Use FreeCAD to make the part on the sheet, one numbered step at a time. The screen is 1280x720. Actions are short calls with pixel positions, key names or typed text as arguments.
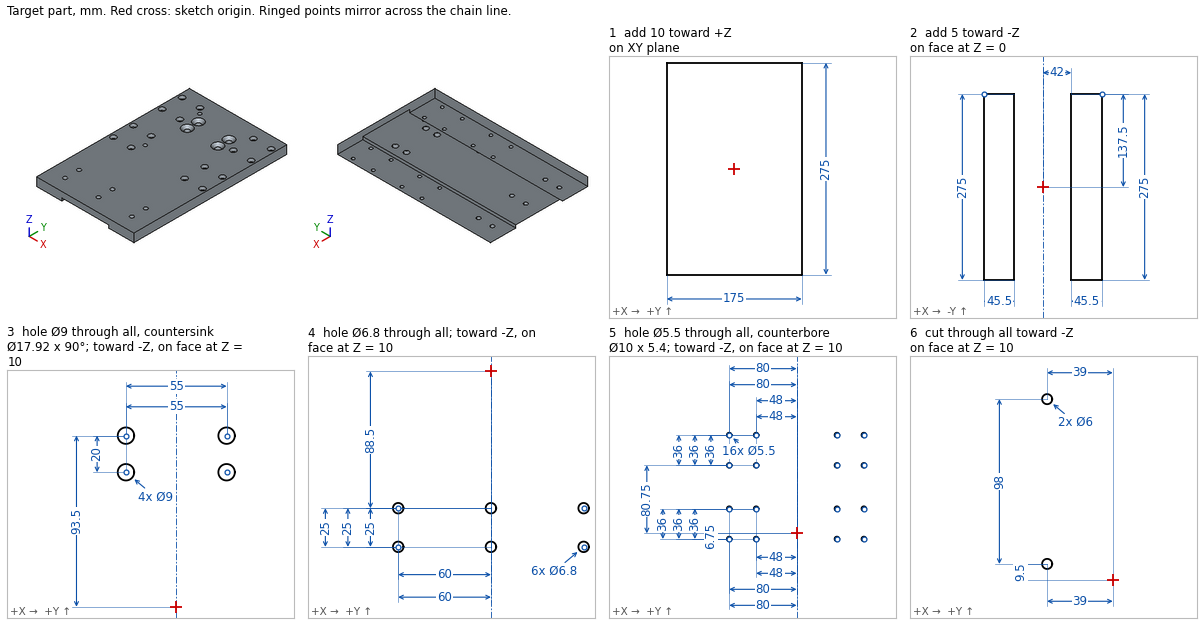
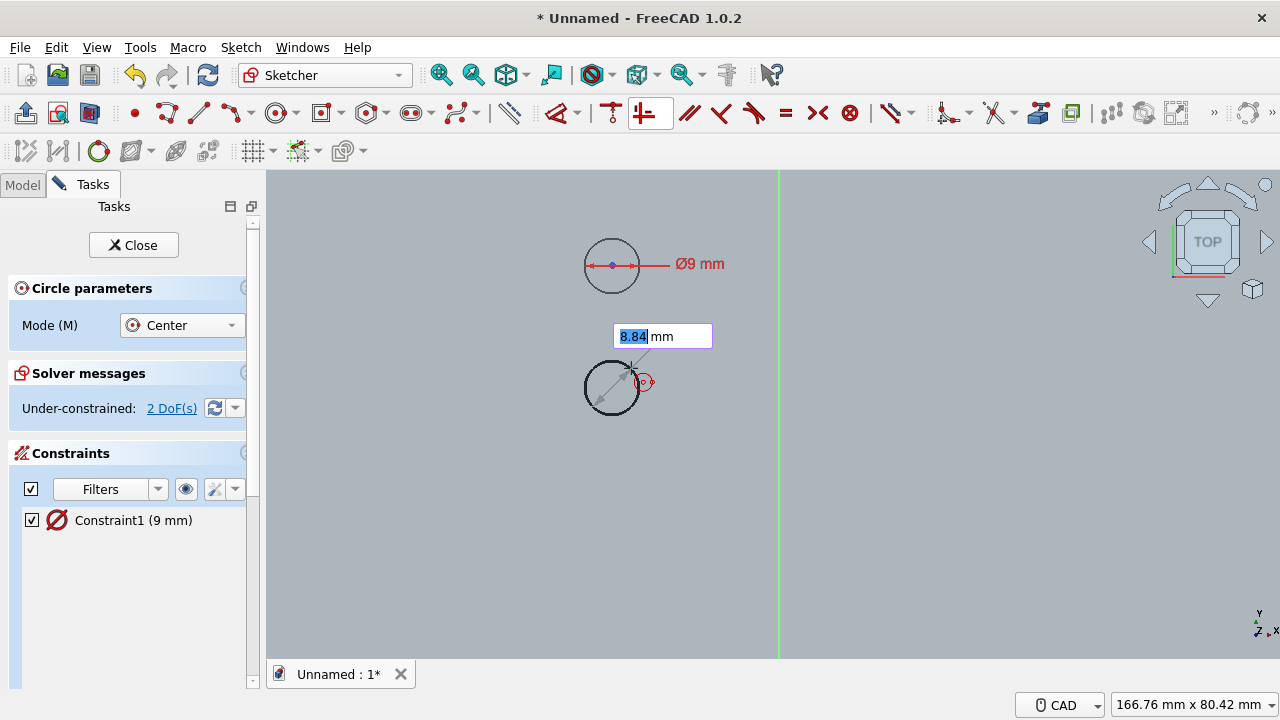
text(9)
key(Return)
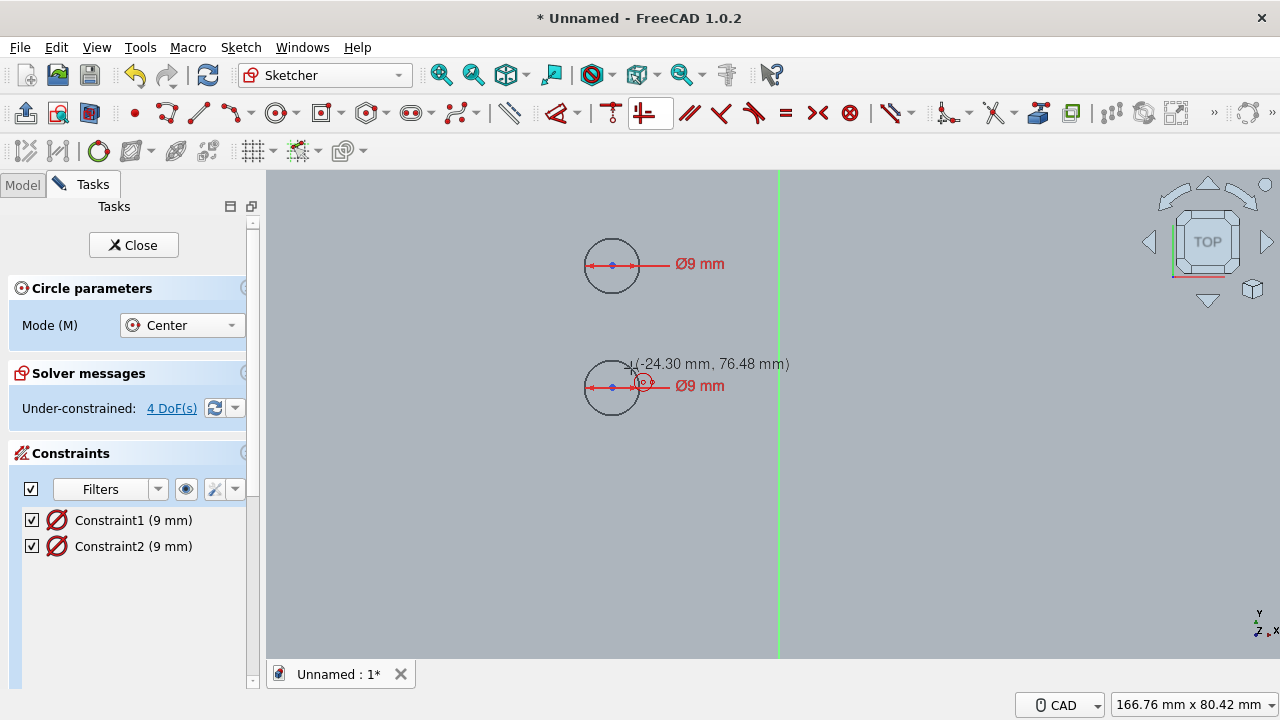
click(946, 265)
move(965, 246)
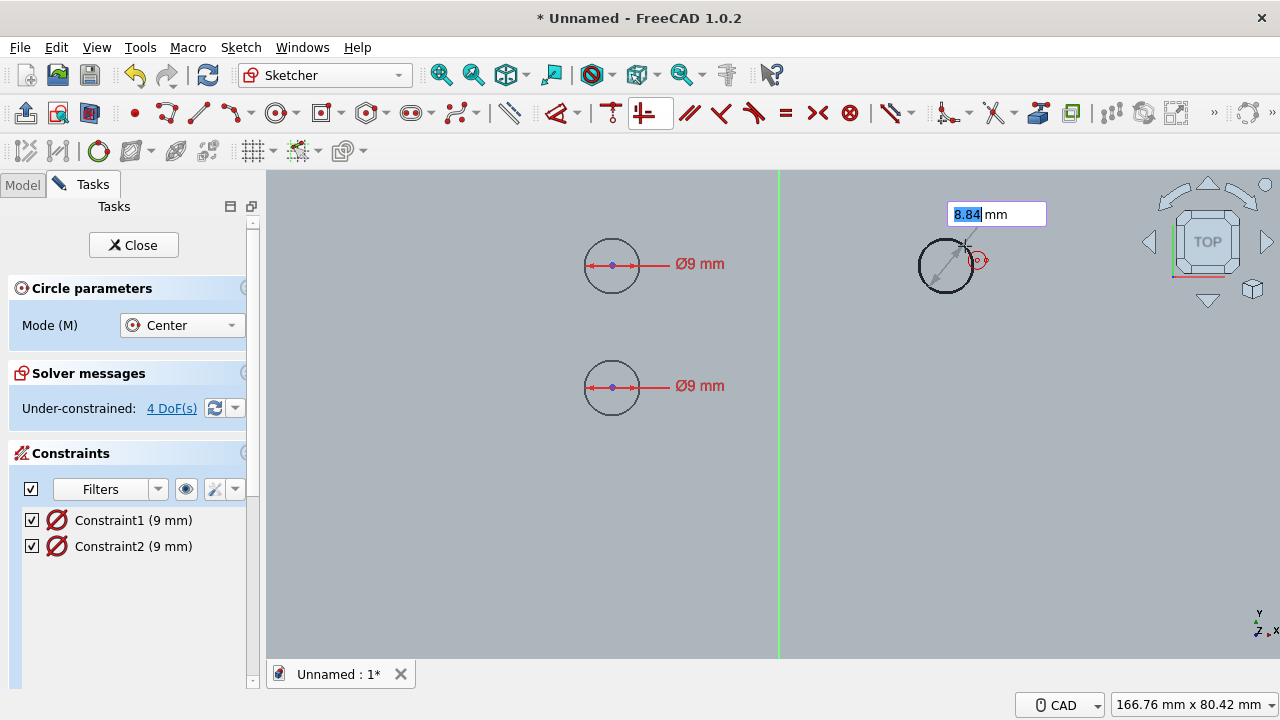
text(9)
key(Return)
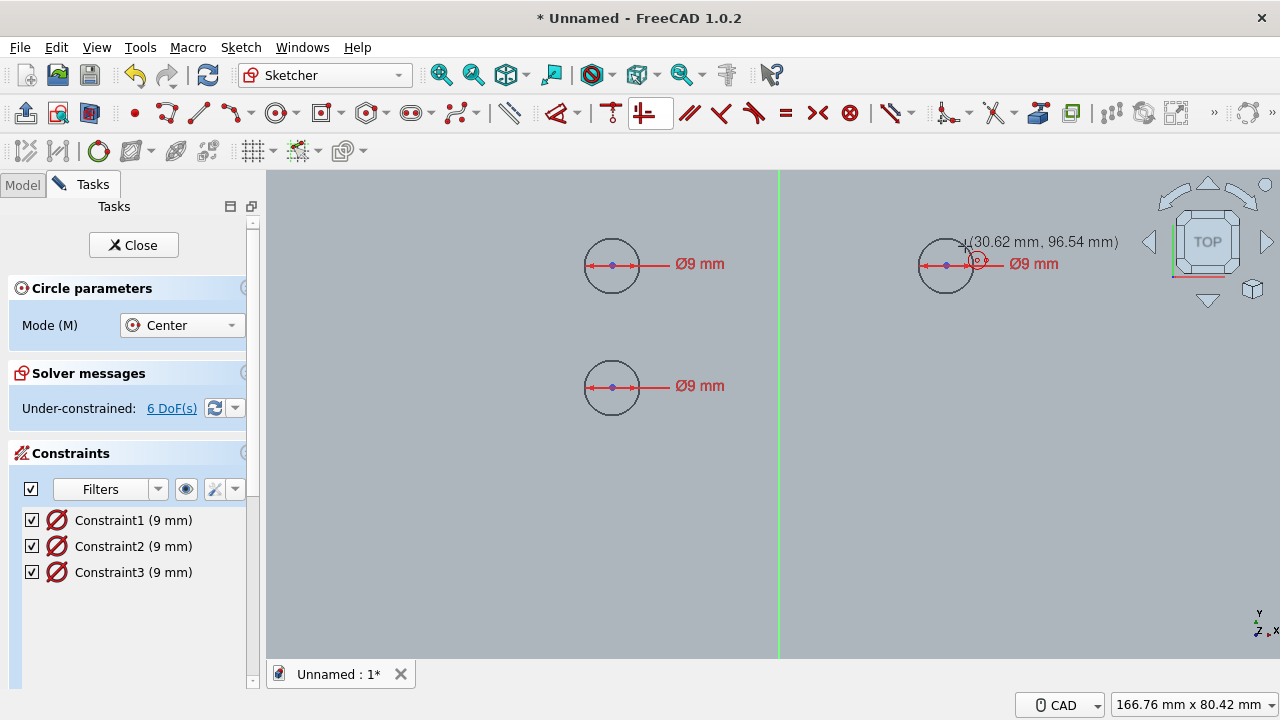
click(946, 387)
move(965, 368)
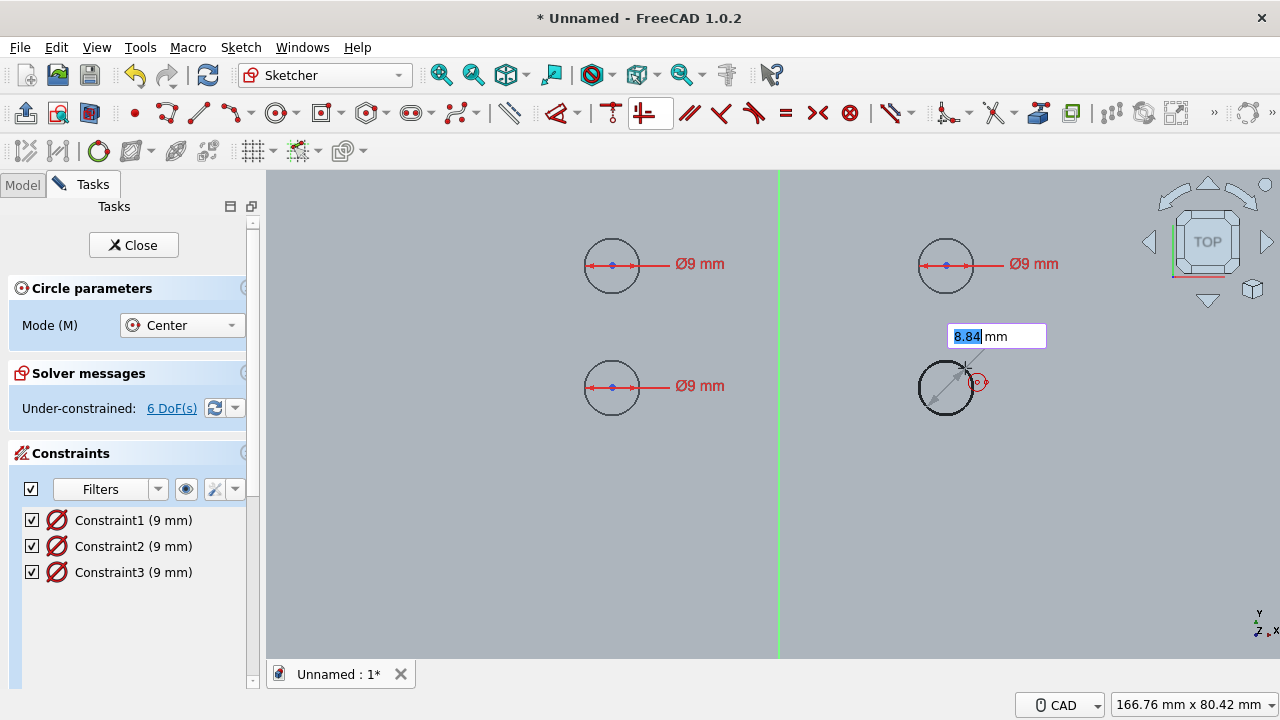
text(9)
key(Return)
key(Escape)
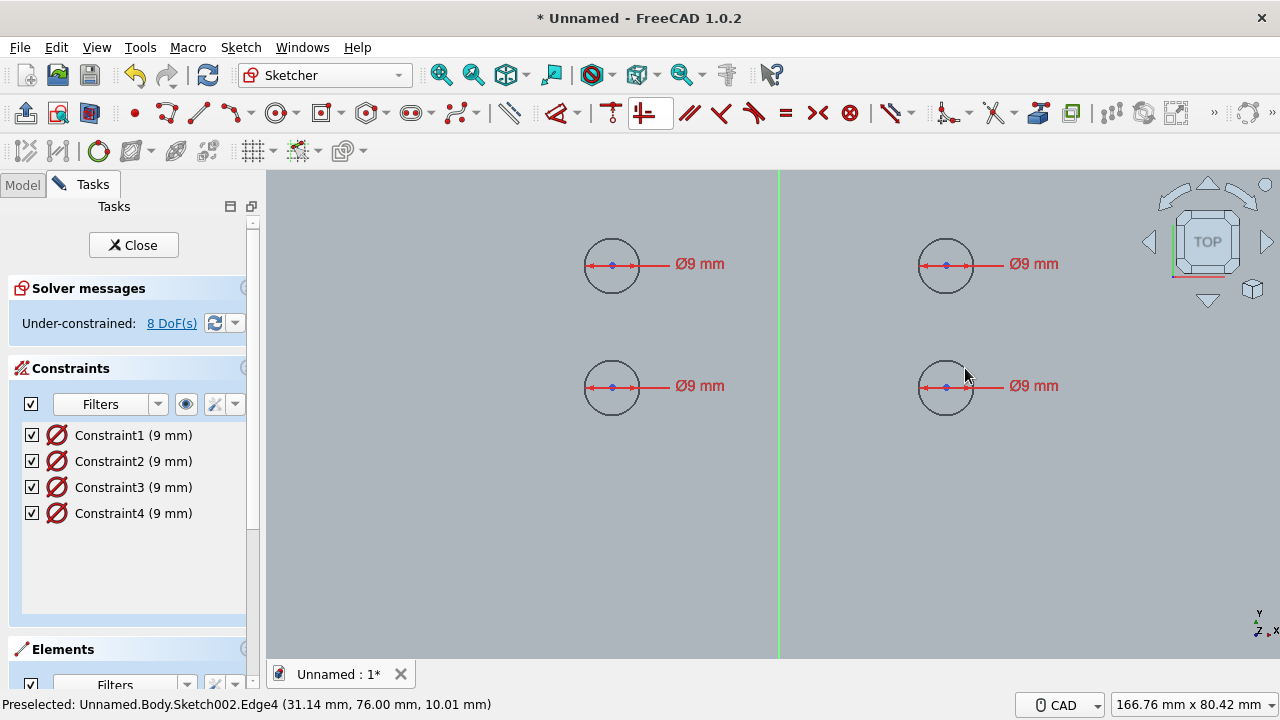
click(612, 266)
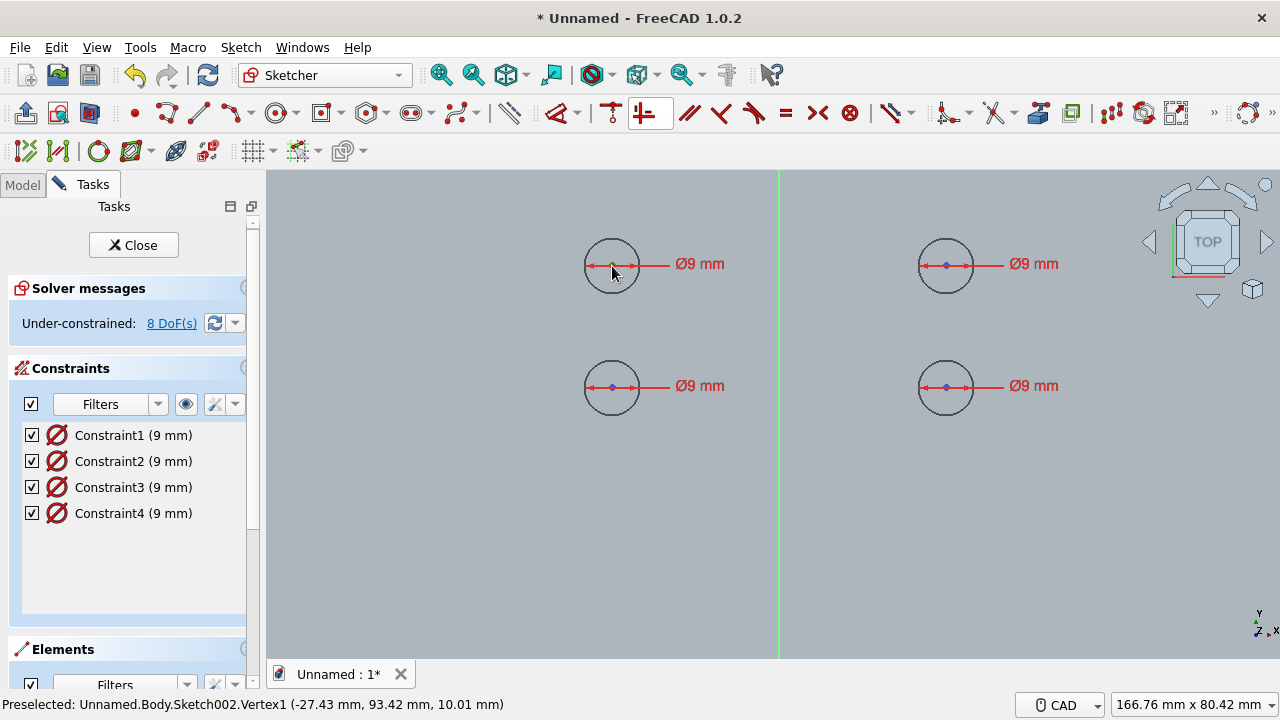
click(946, 266)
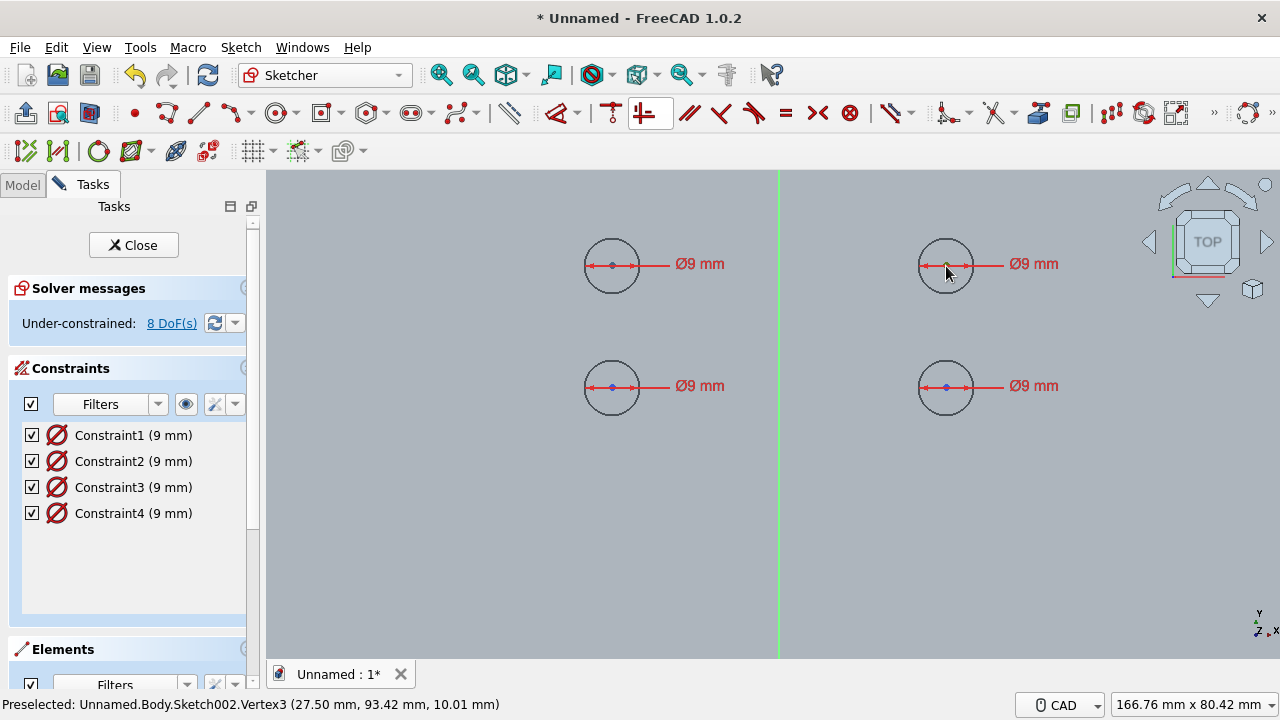
click(779, 600)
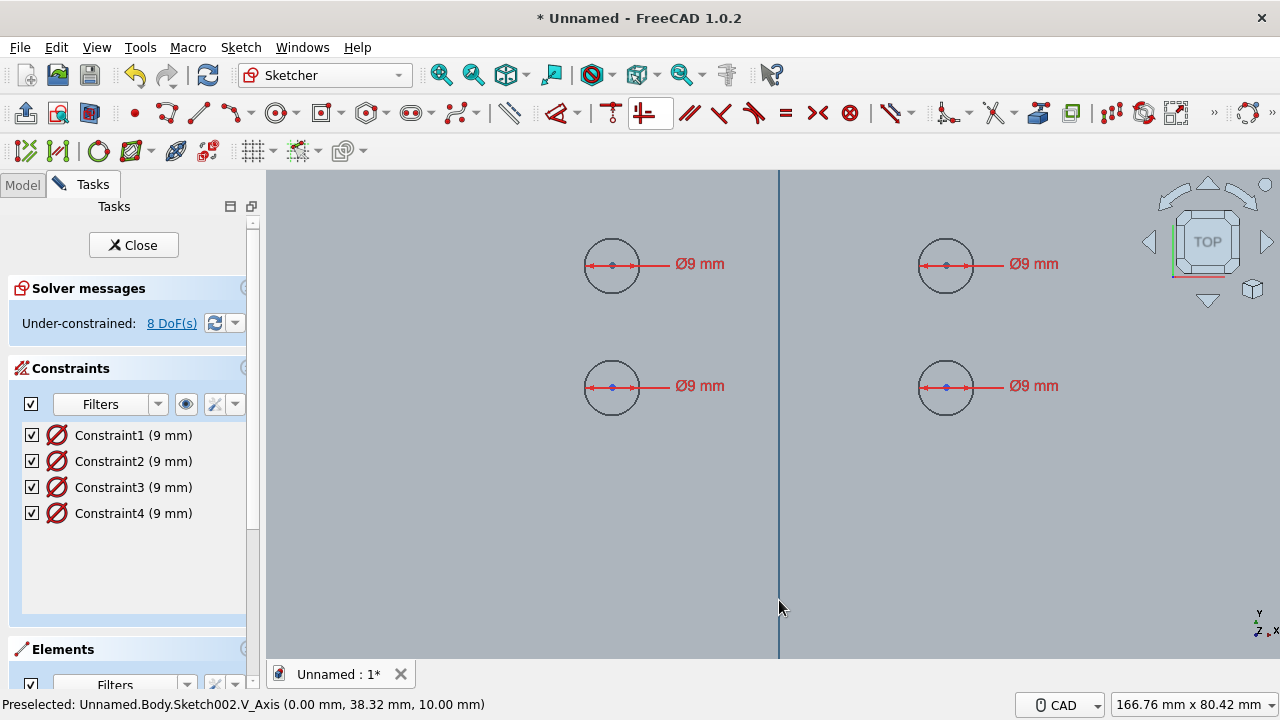
click(818, 114)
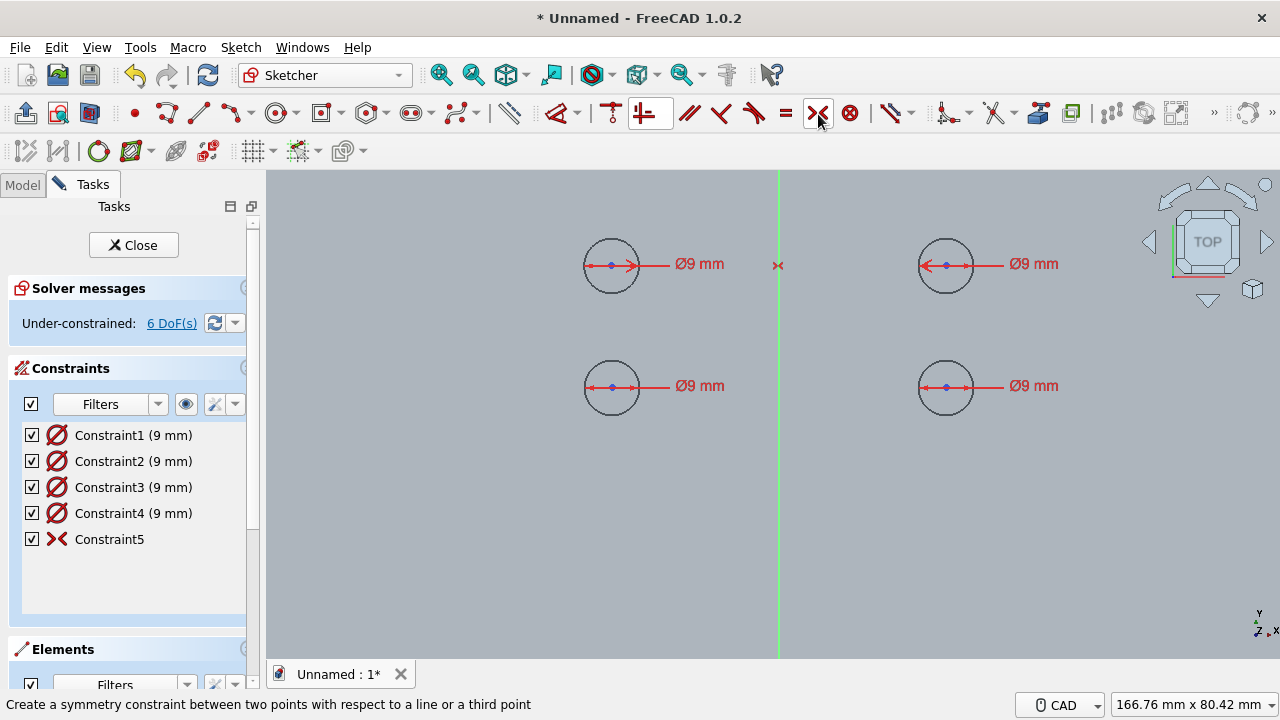
click(612, 388)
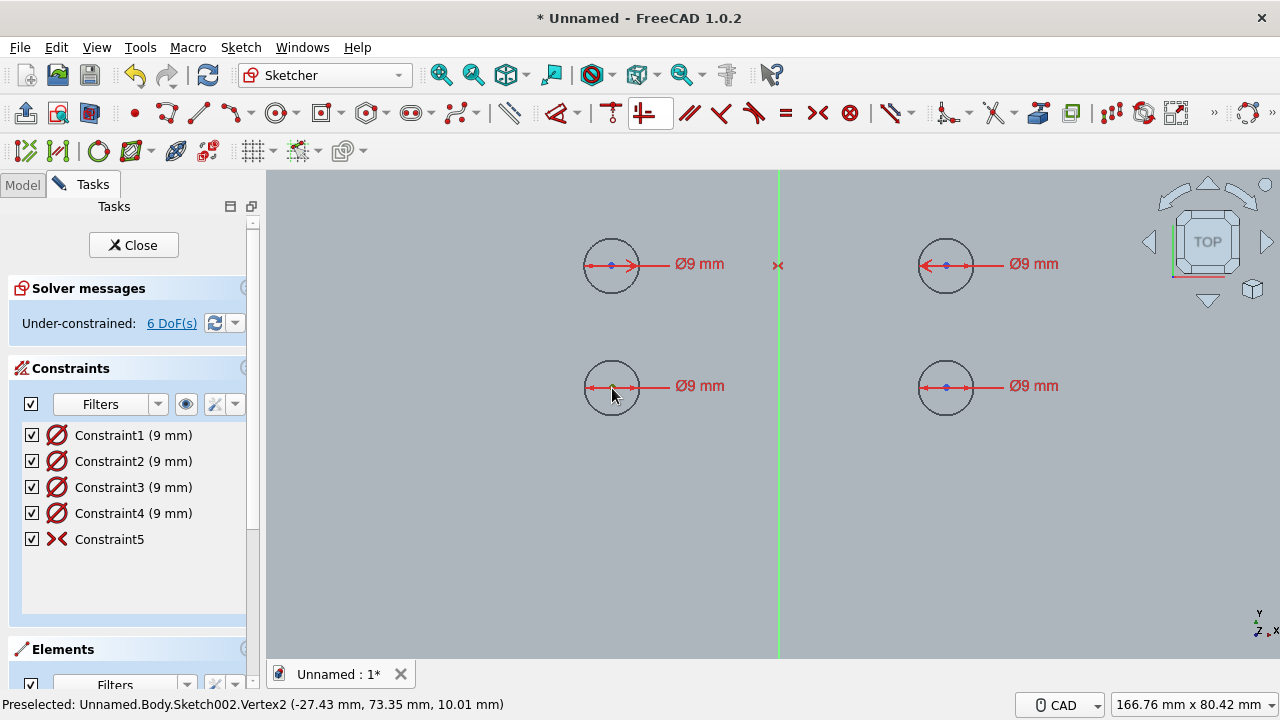
click(946, 388)